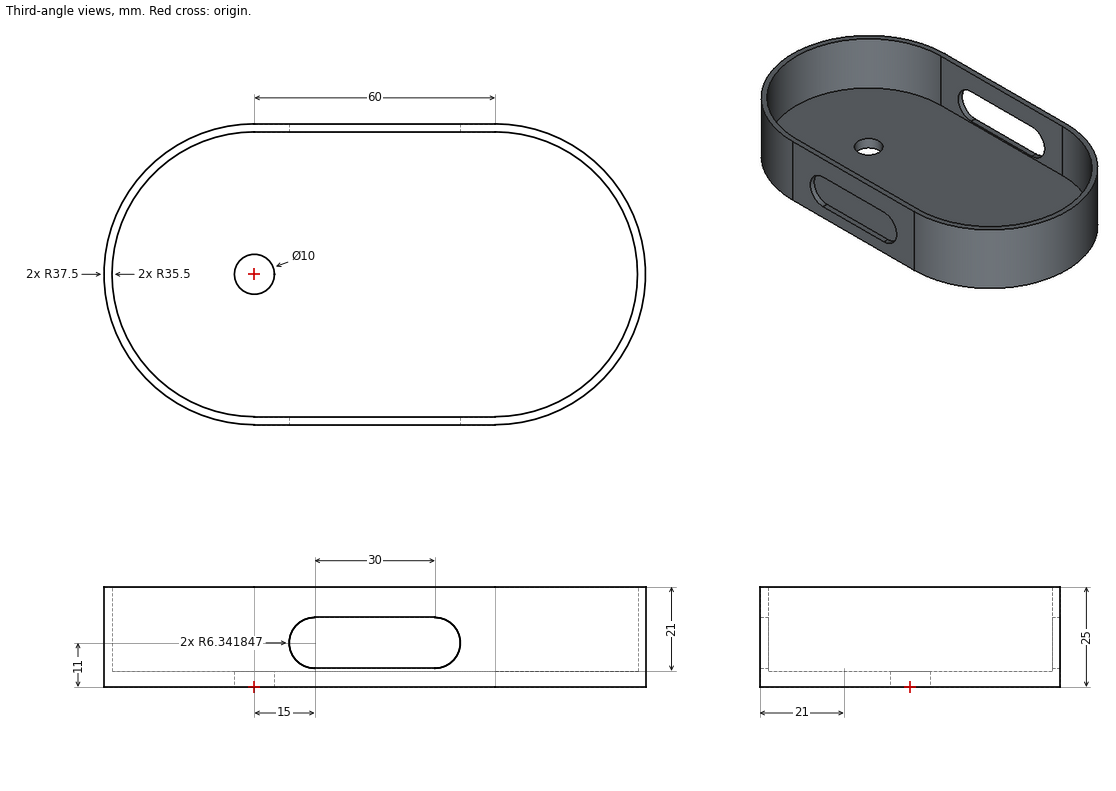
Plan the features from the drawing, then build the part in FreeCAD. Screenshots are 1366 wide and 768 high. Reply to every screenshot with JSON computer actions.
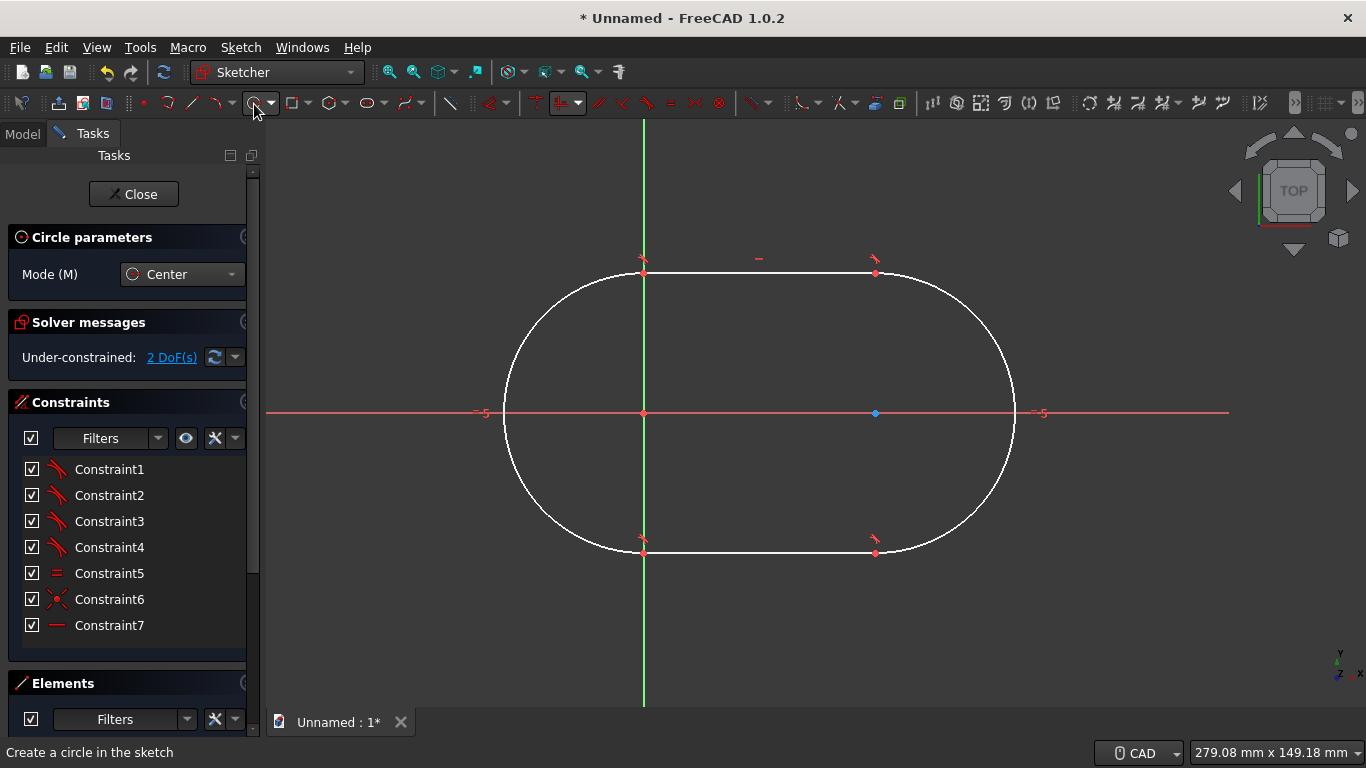
{"action": "left_click", "coordinate": [644, 413]}
{"action": "left_click", "coordinate": [658, 399]}
{"action": "key", "text": "Escape"}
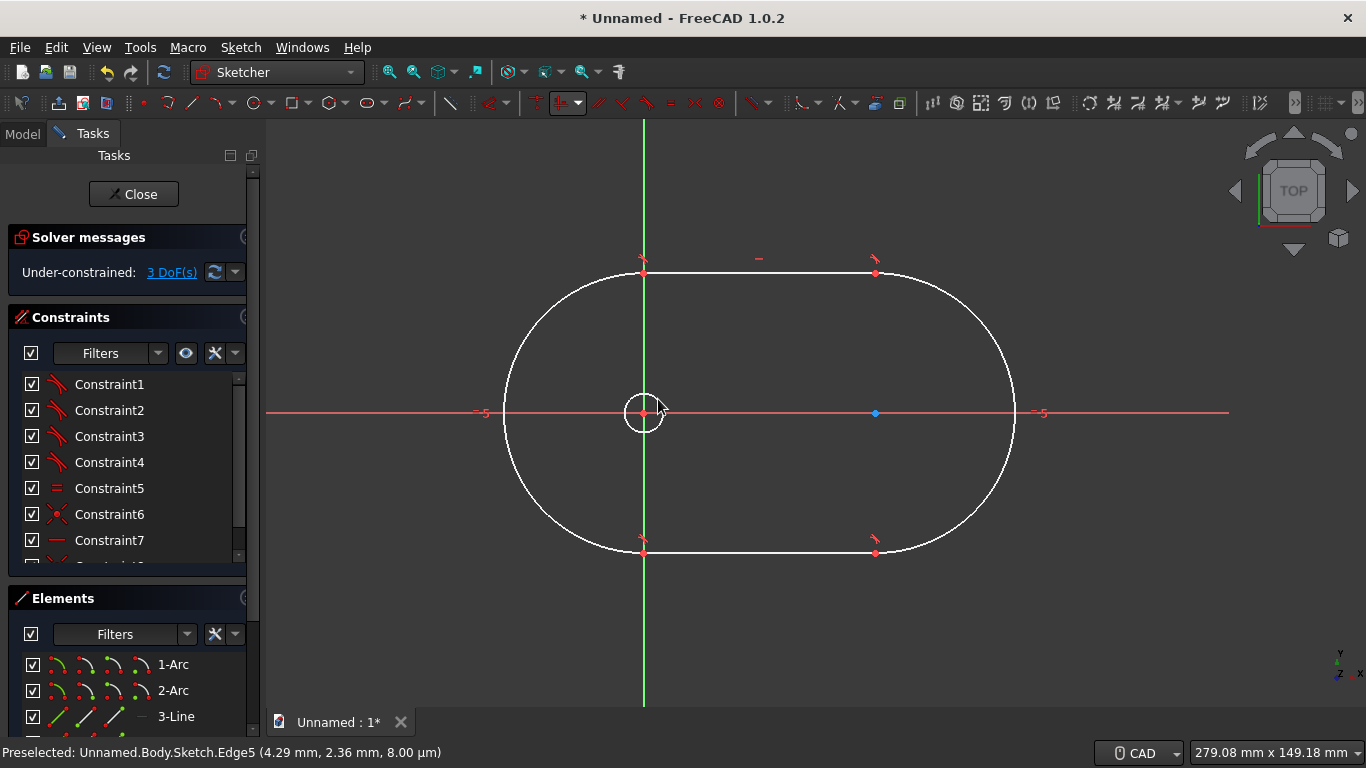
{"action": "left_click", "coordinate": [490, 104]}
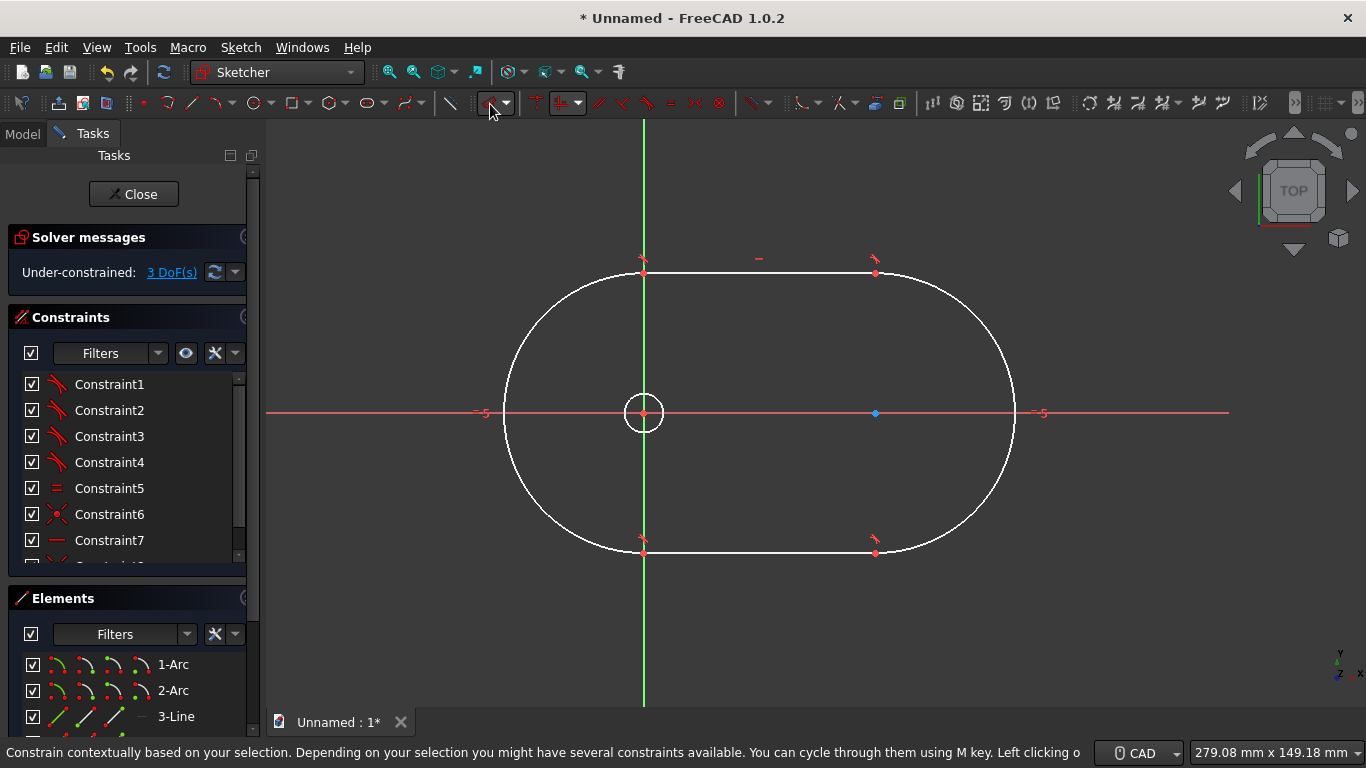
{"action": "left_click", "coordinate": [531, 331]}
{"action": "left_click", "coordinate": [505, 312]}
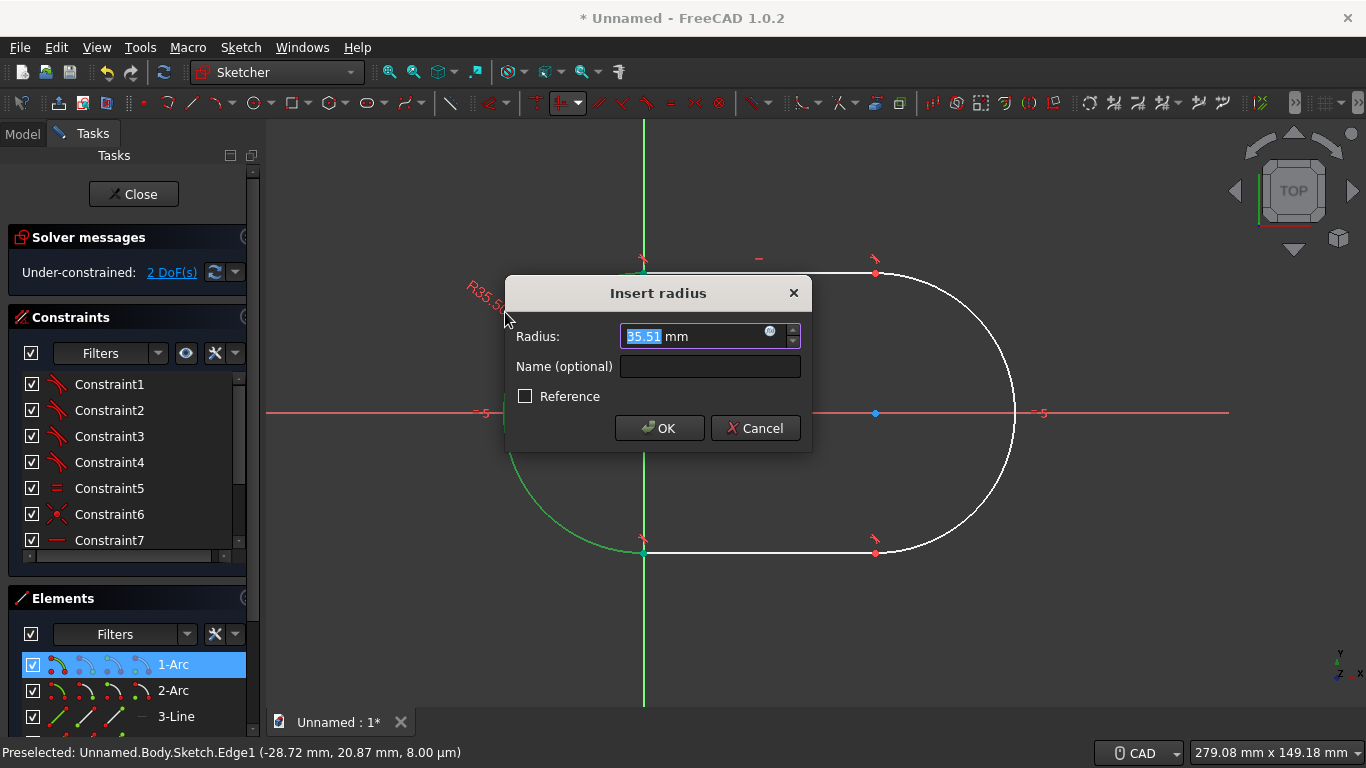
{"action": "type", "text": "37.5"}
{"action": "key", "text": "Return"}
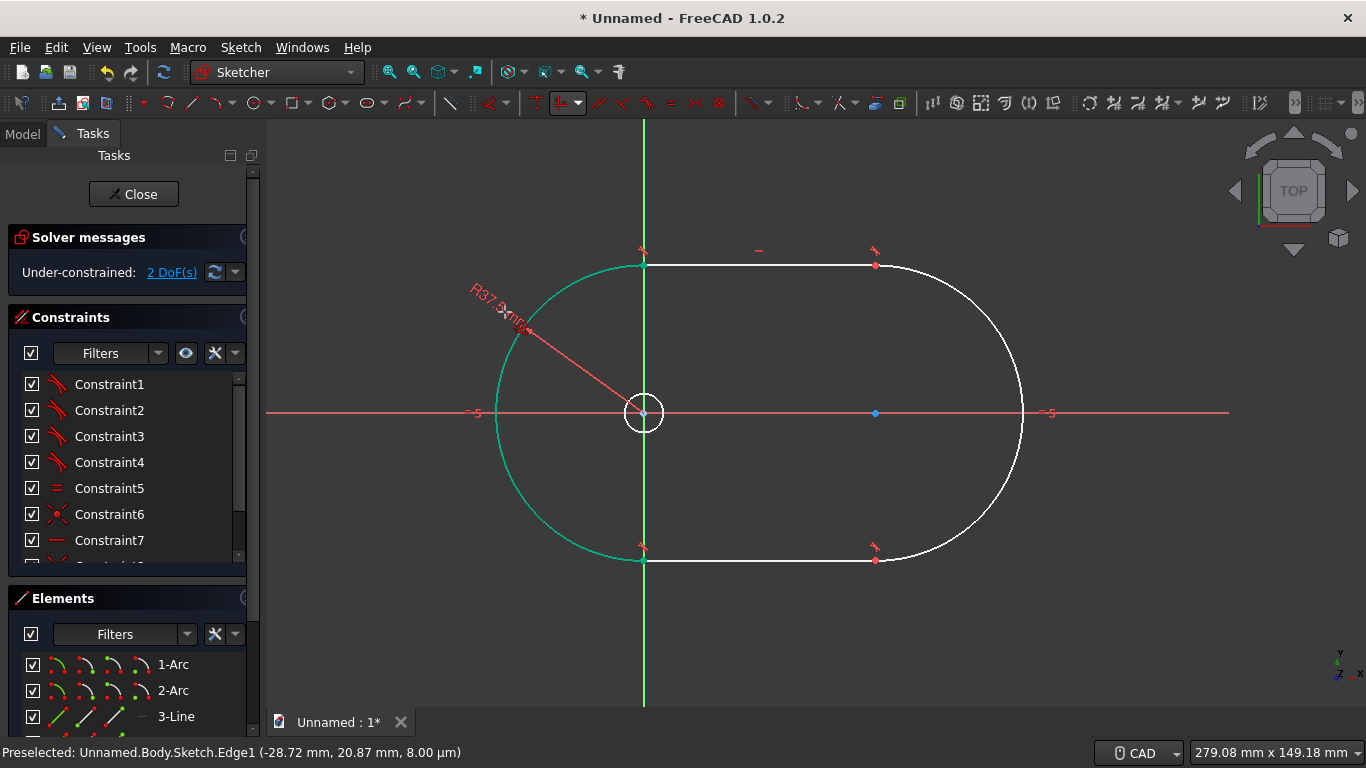
{"action": "left_click", "coordinate": [658, 399]}
{"action": "left_click", "coordinate": [681, 376]}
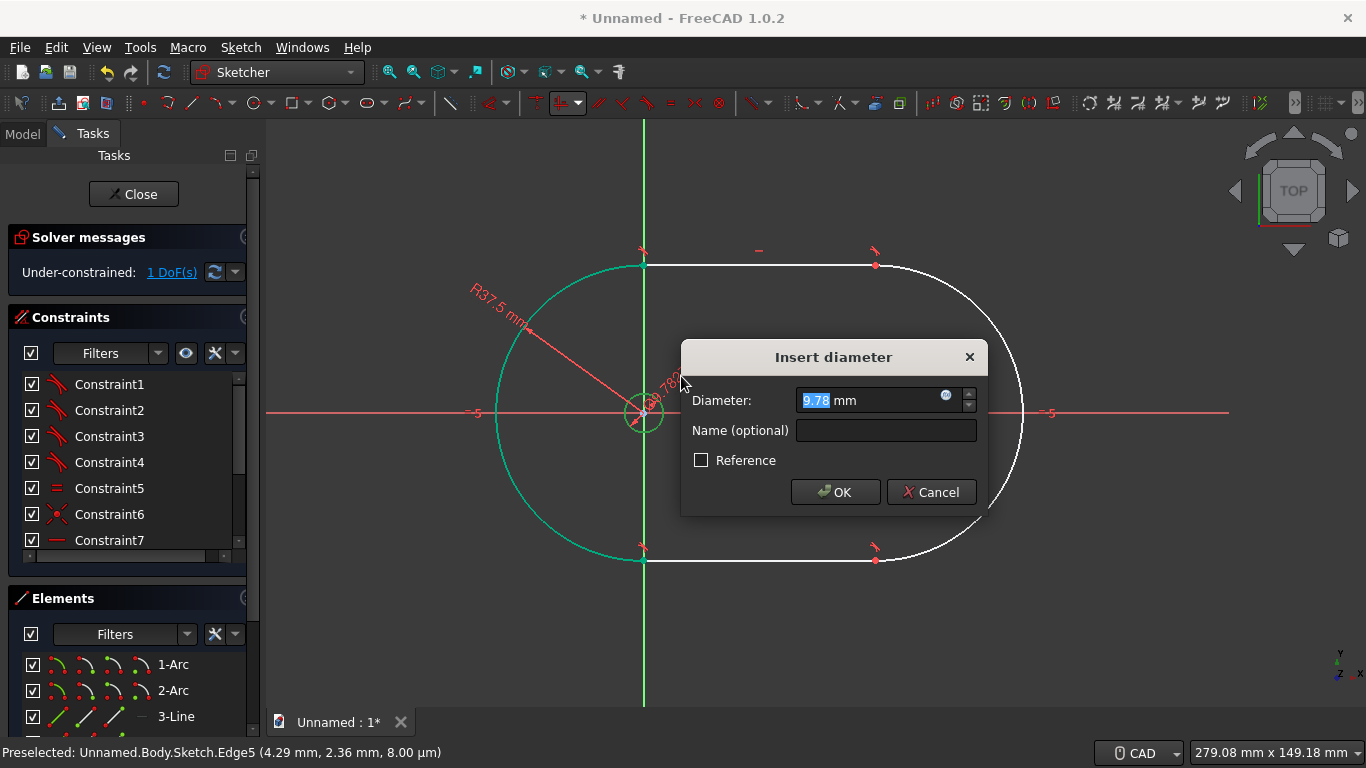
{"action": "type", "text": "10"}
{"action": "key", "text": "Return"}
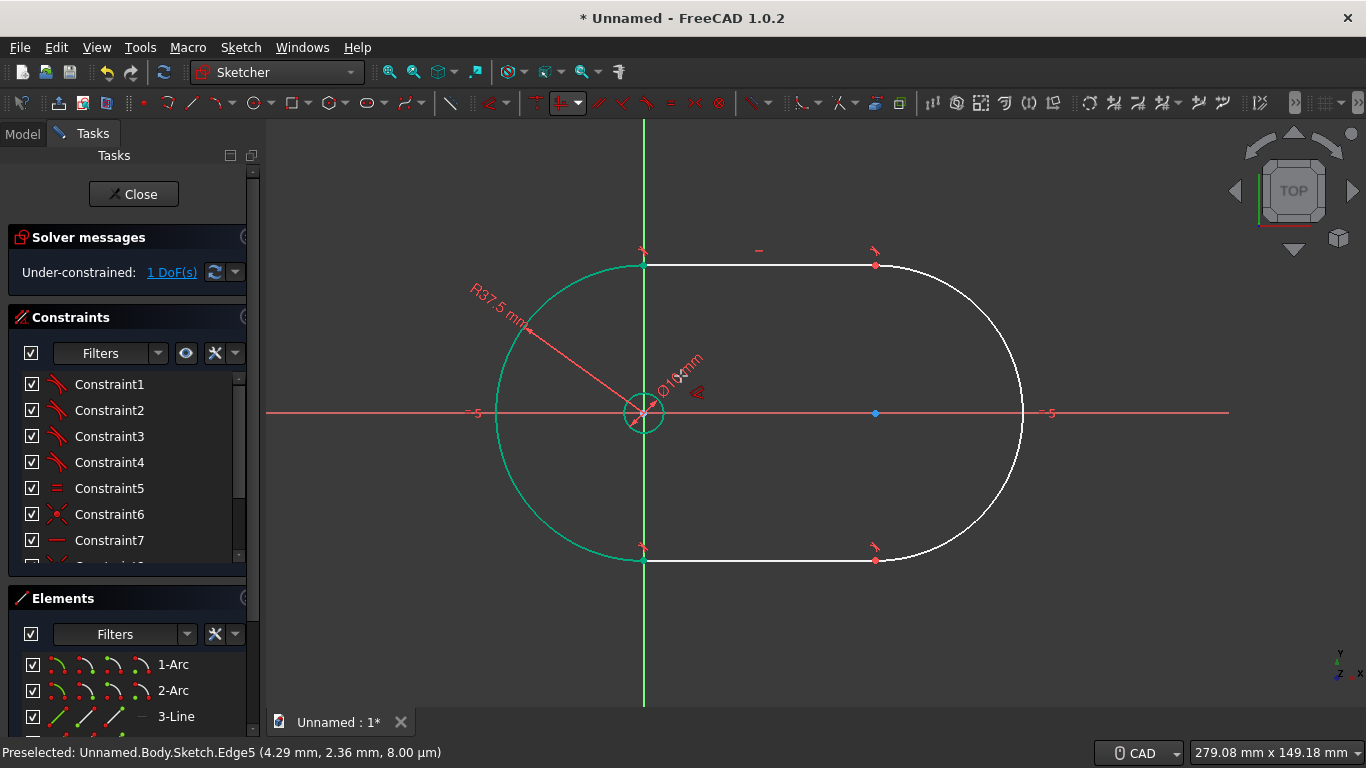
{"action": "left_click", "coordinate": [713, 265]}
{"action": "left_click", "coordinate": [759, 231]}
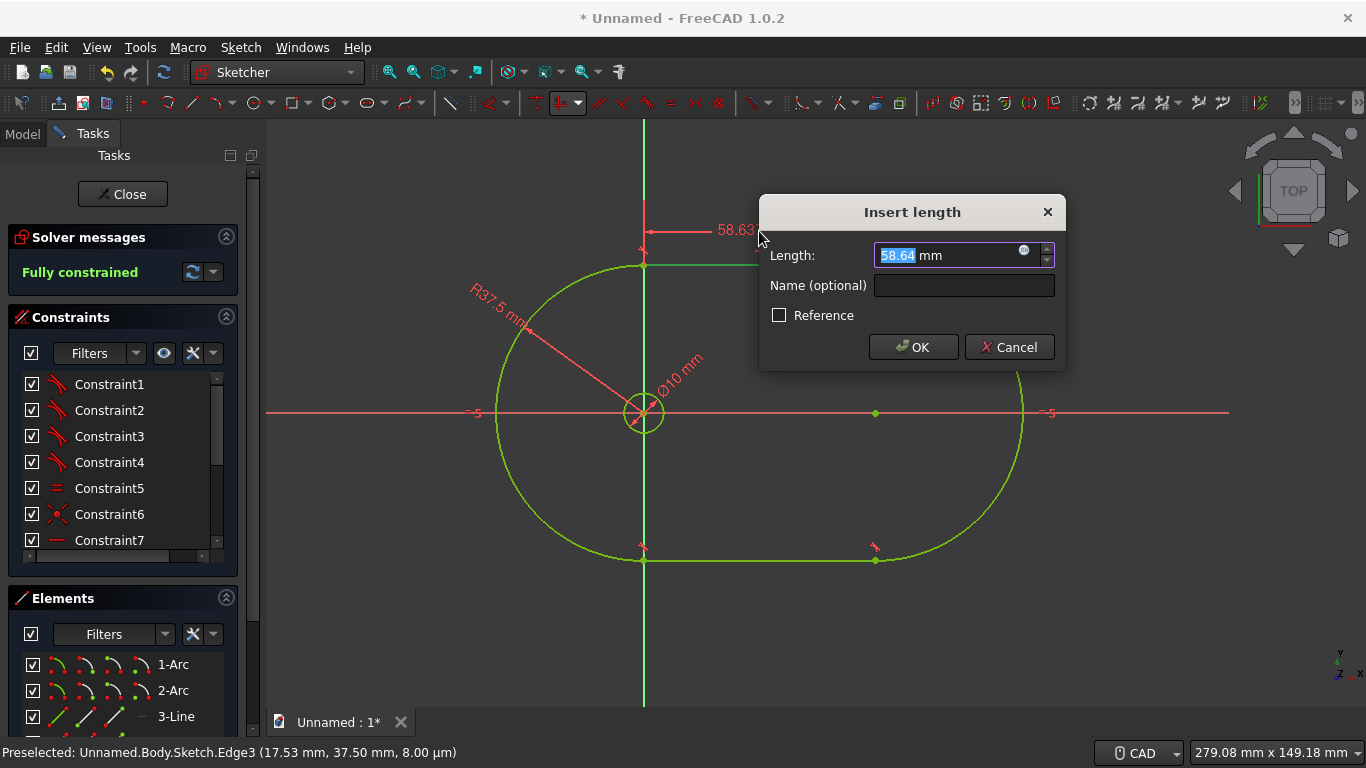
{"action": "type", "text": "60"}
{"action": "key", "text": "Return"}
{"action": "key", "text": "Escape"}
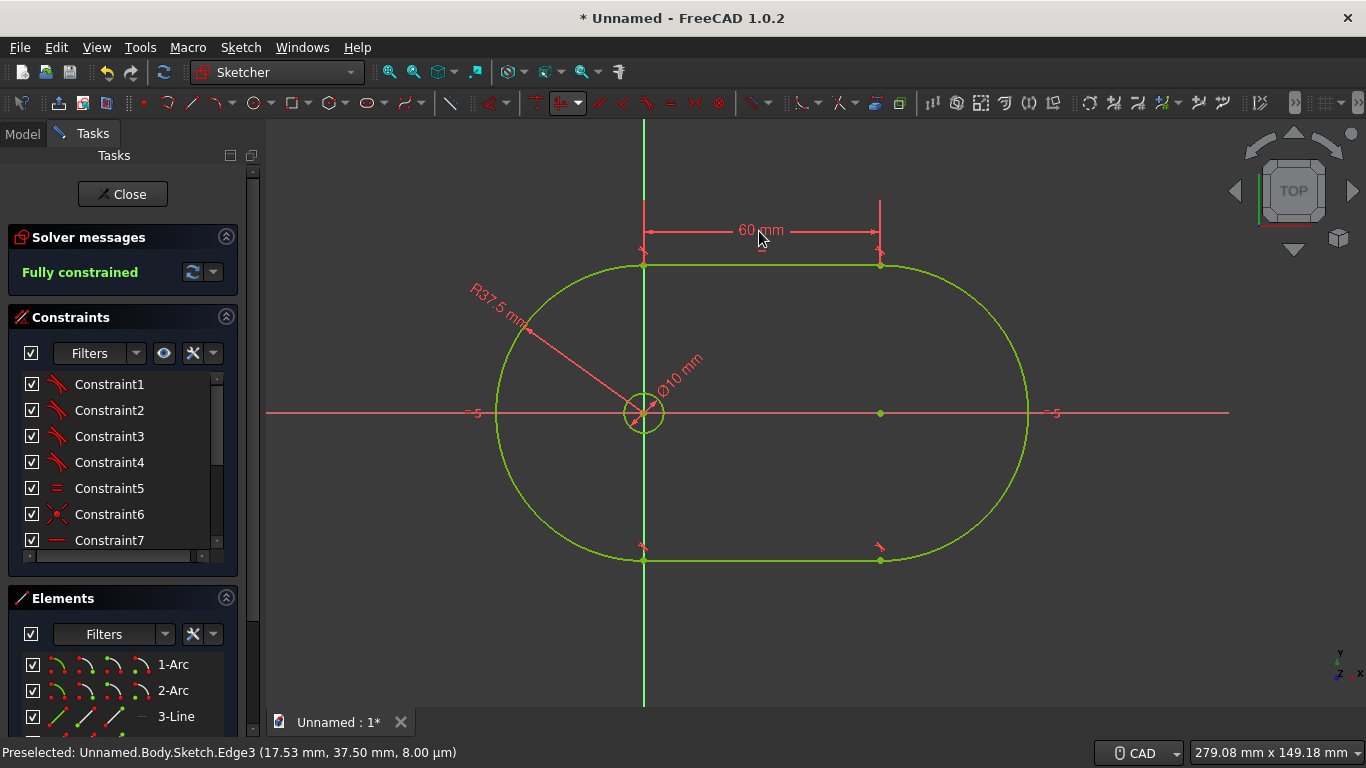
{"action": "left_click", "coordinate": [123, 194]}